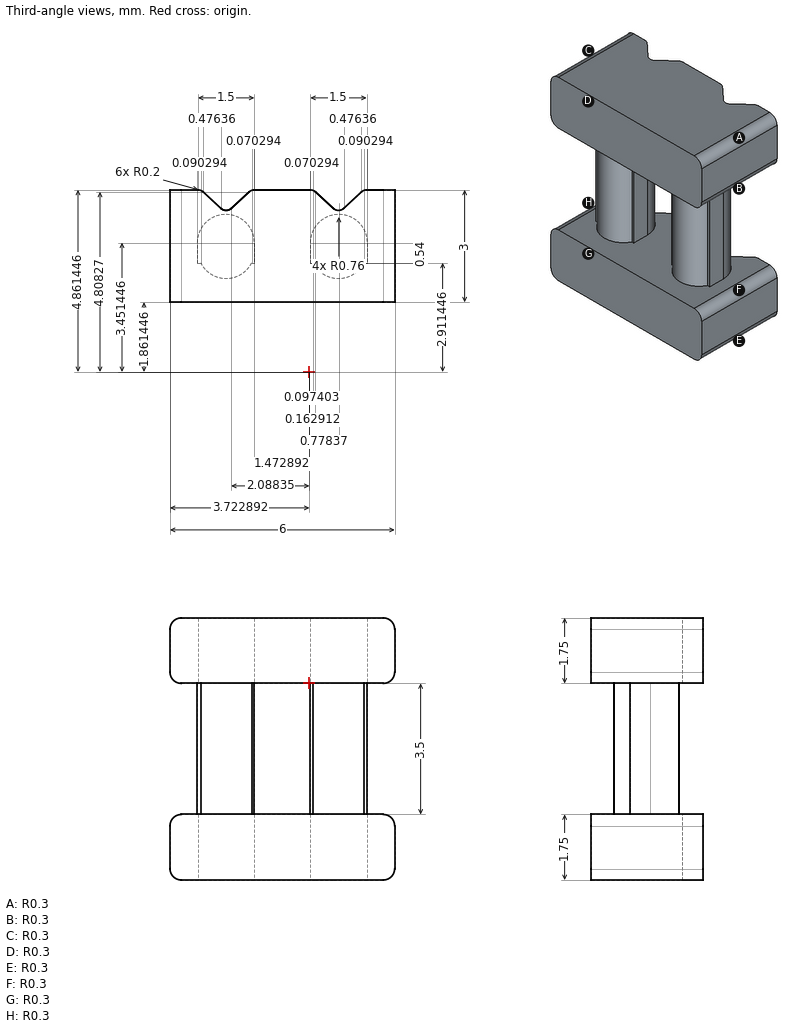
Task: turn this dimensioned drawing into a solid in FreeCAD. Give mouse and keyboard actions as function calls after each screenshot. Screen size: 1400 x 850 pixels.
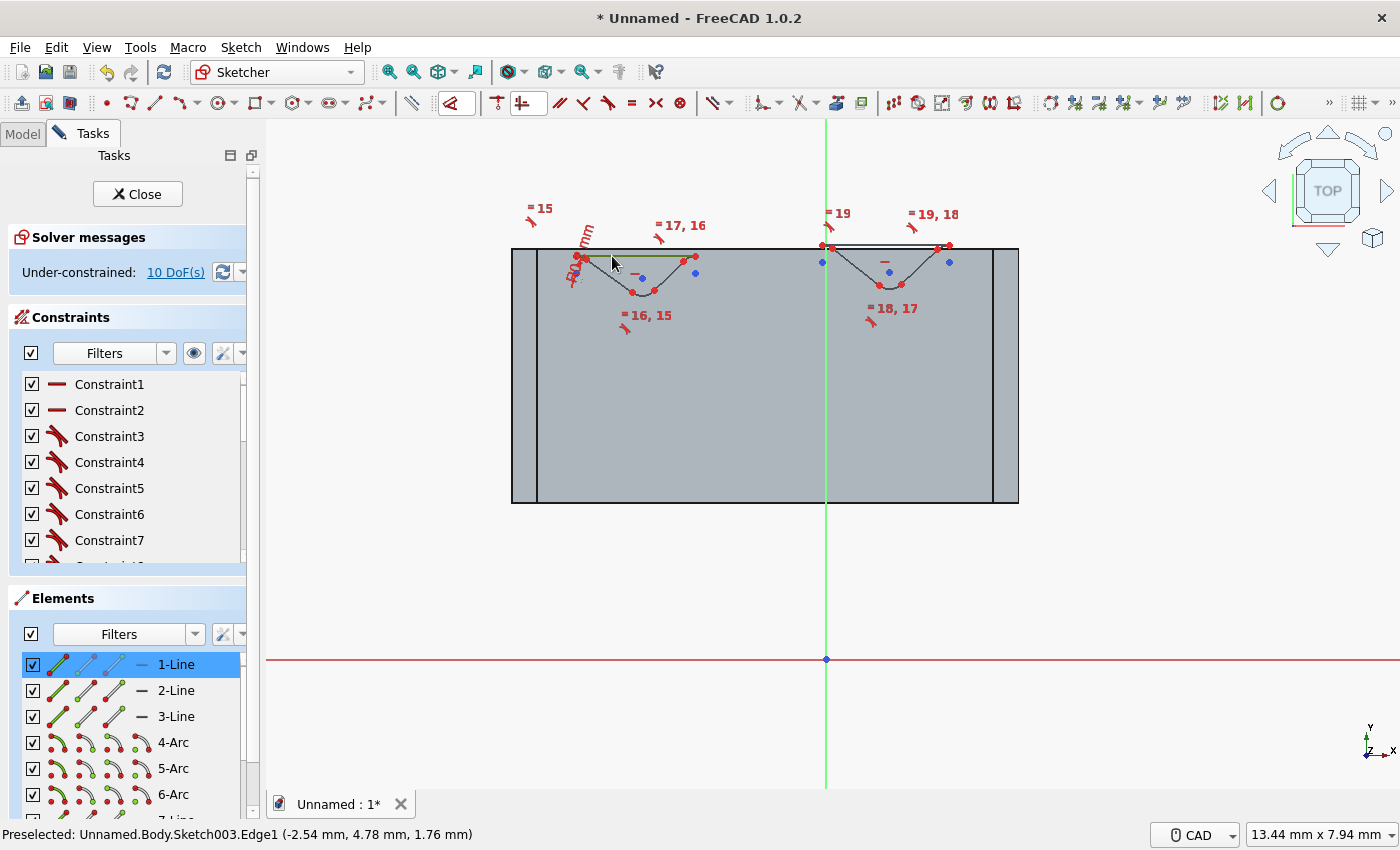
click(470, 104)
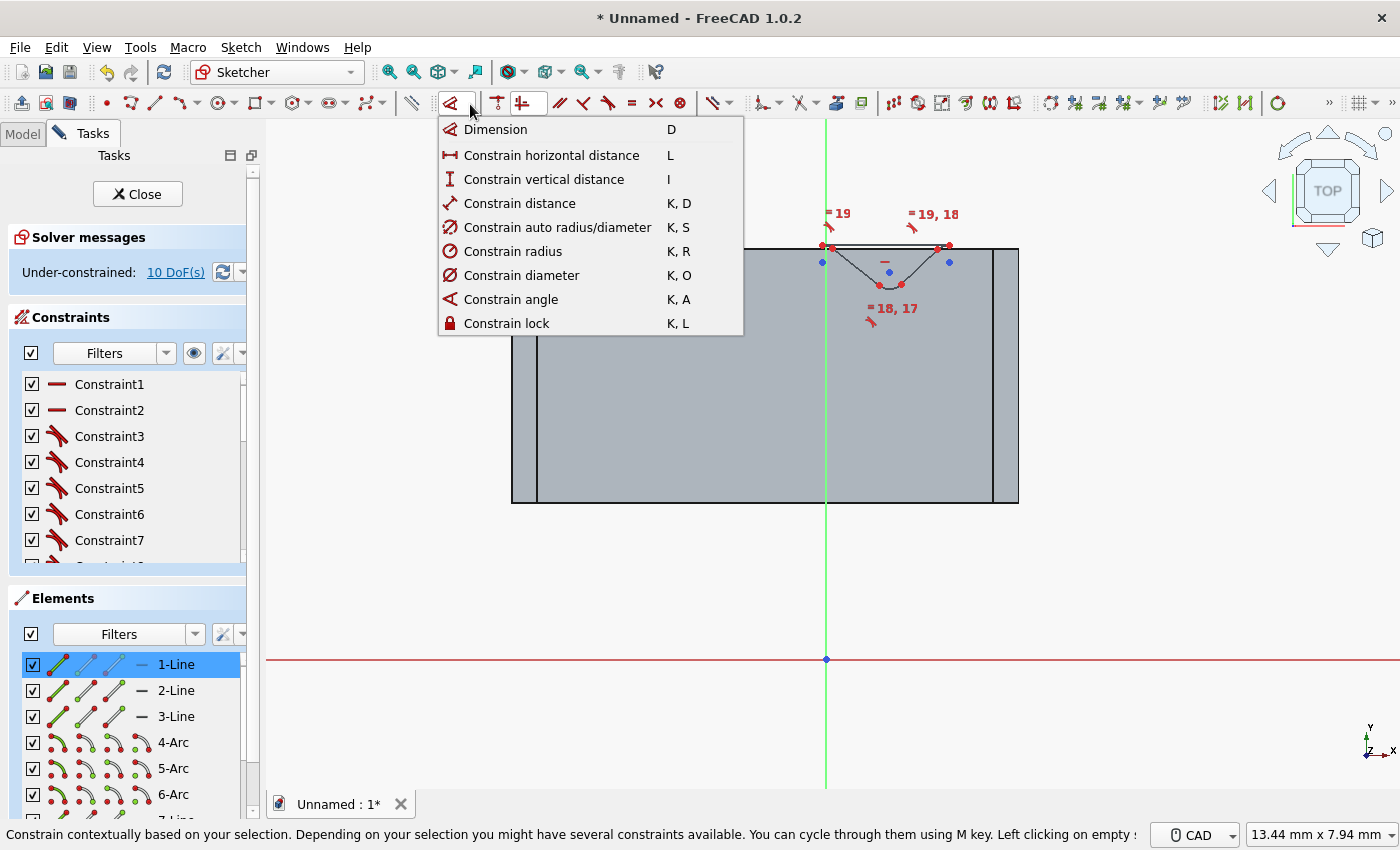
click(591, 155)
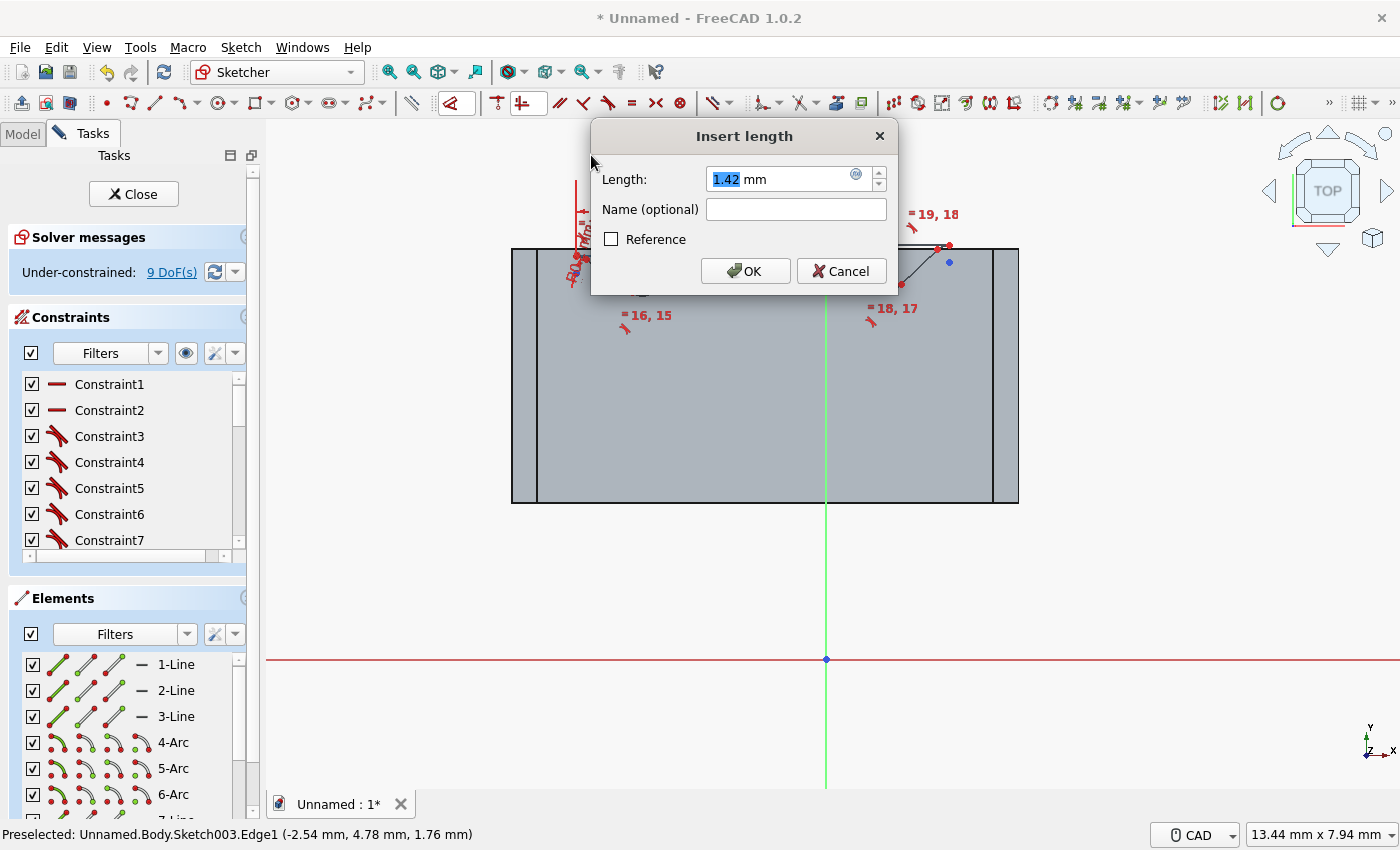
text(1.5)
key(Return)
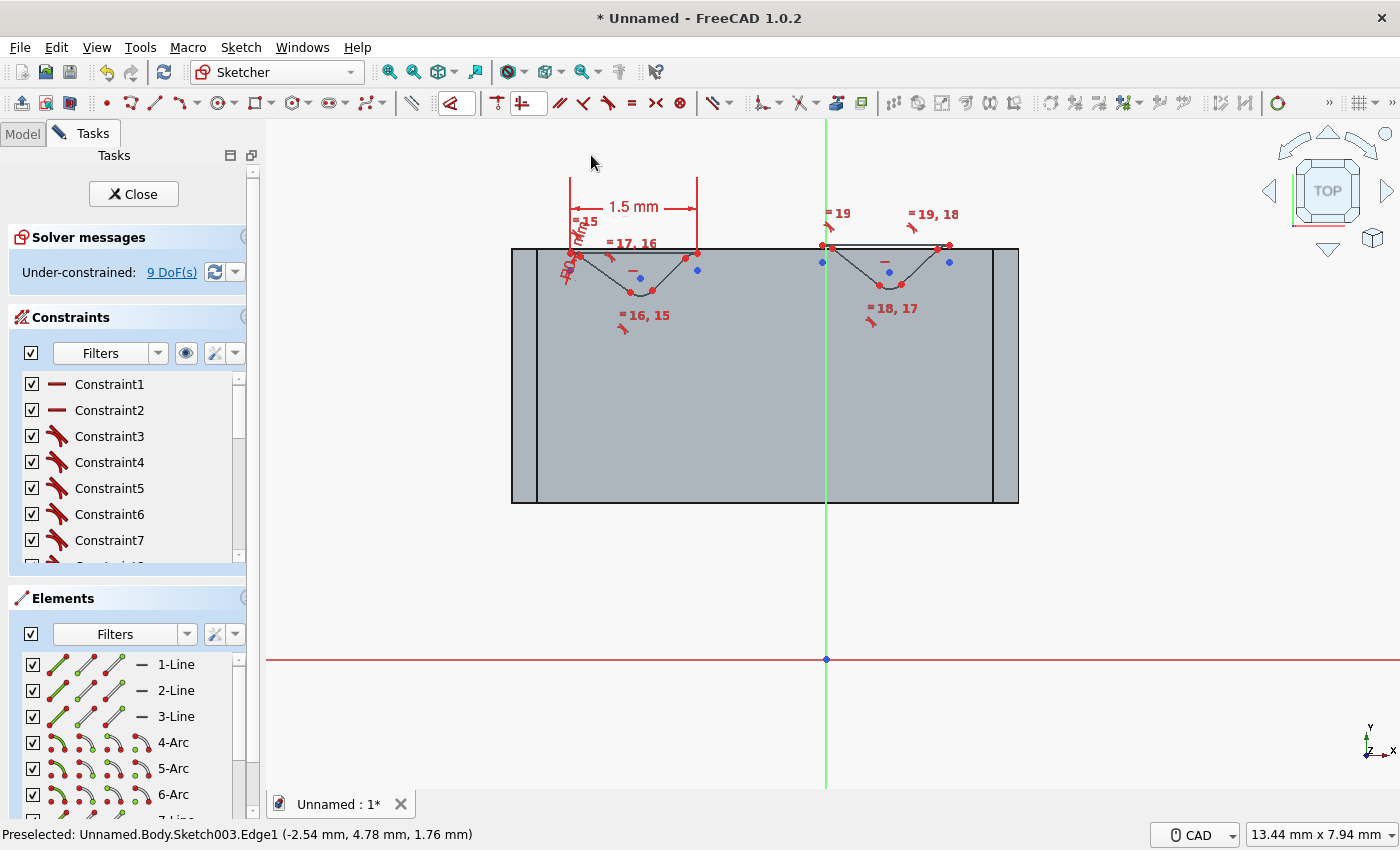
click(911, 245)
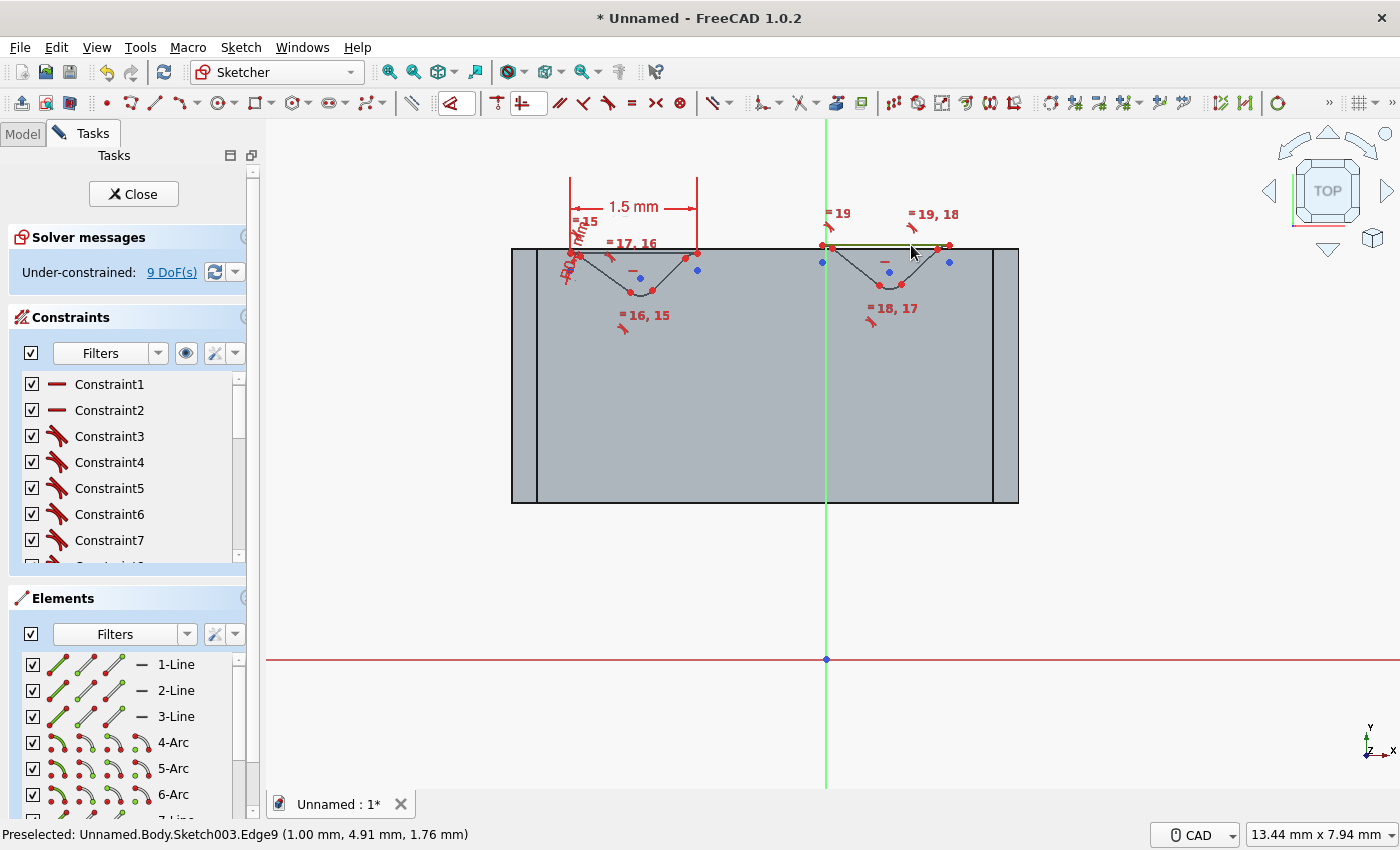
key(l)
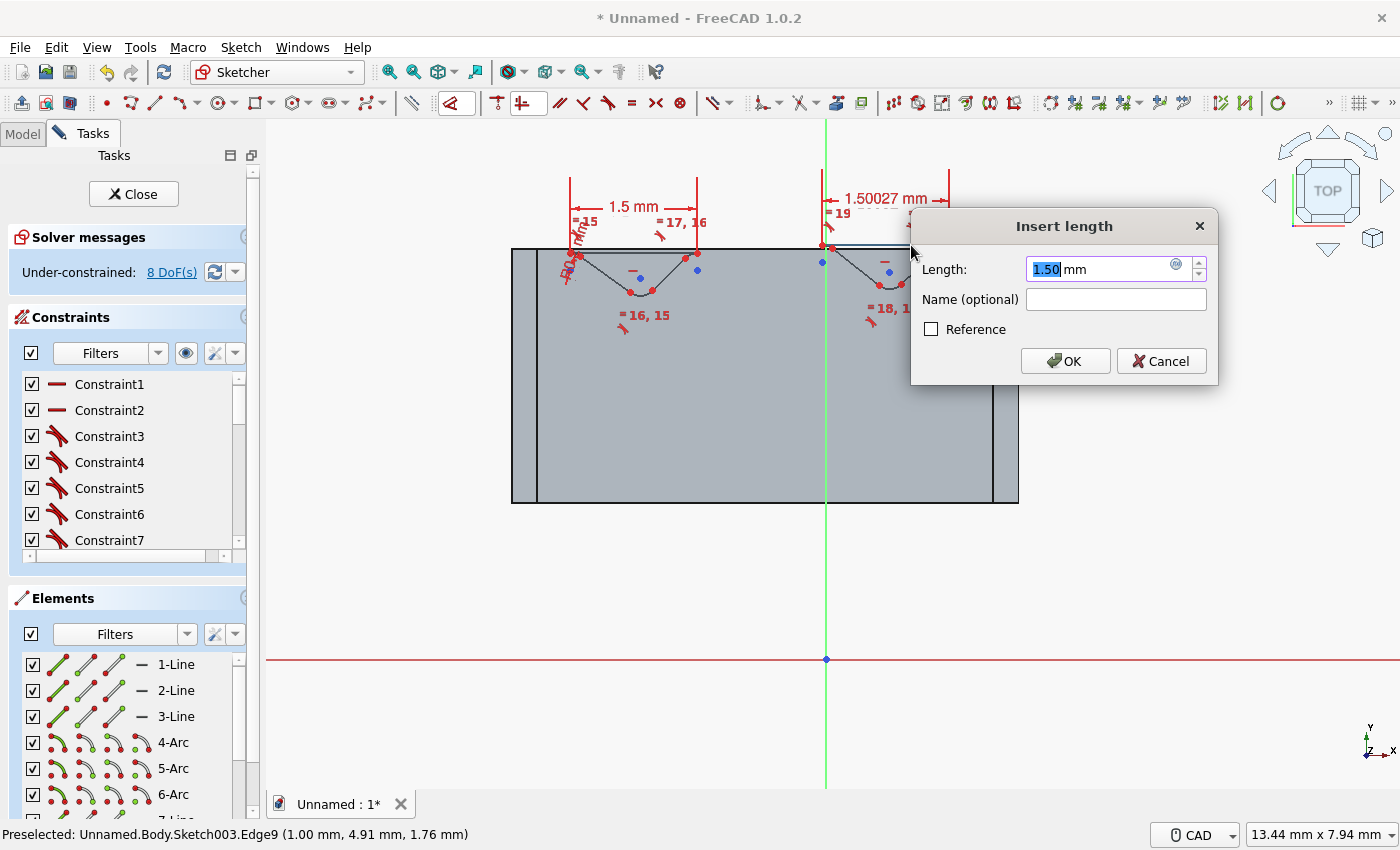
text(1.5)
key(Return)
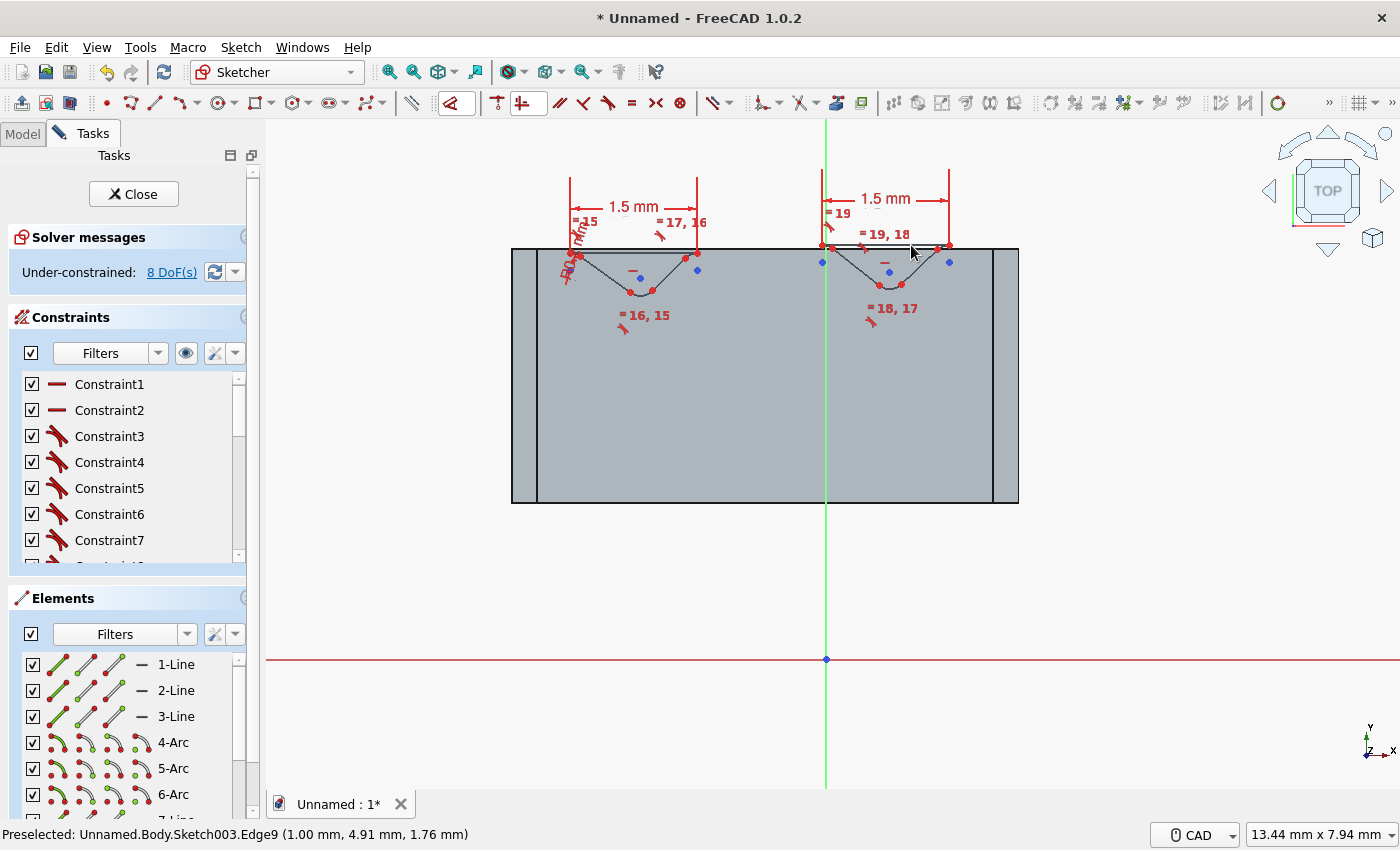
click(652, 291)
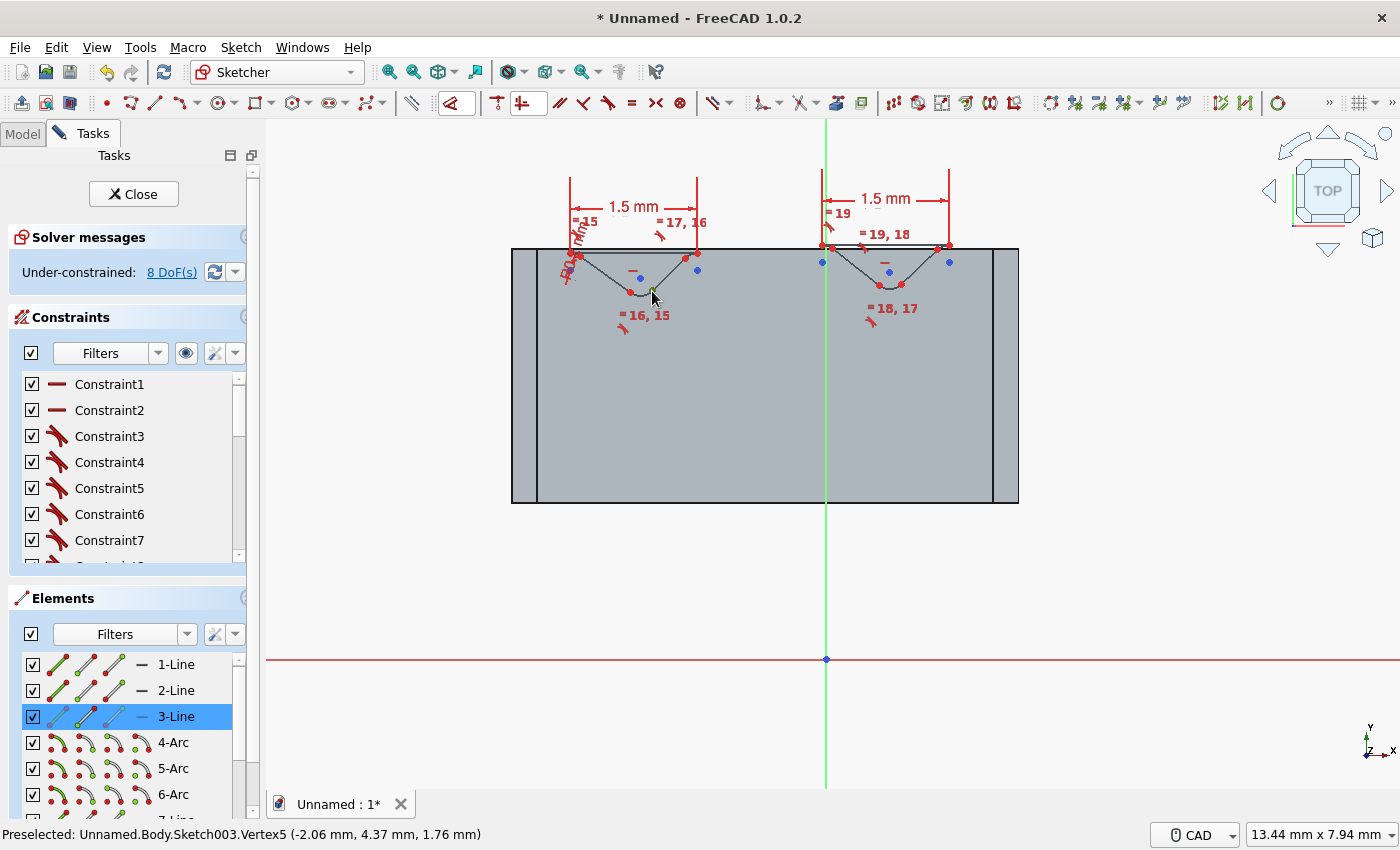
click(470, 104)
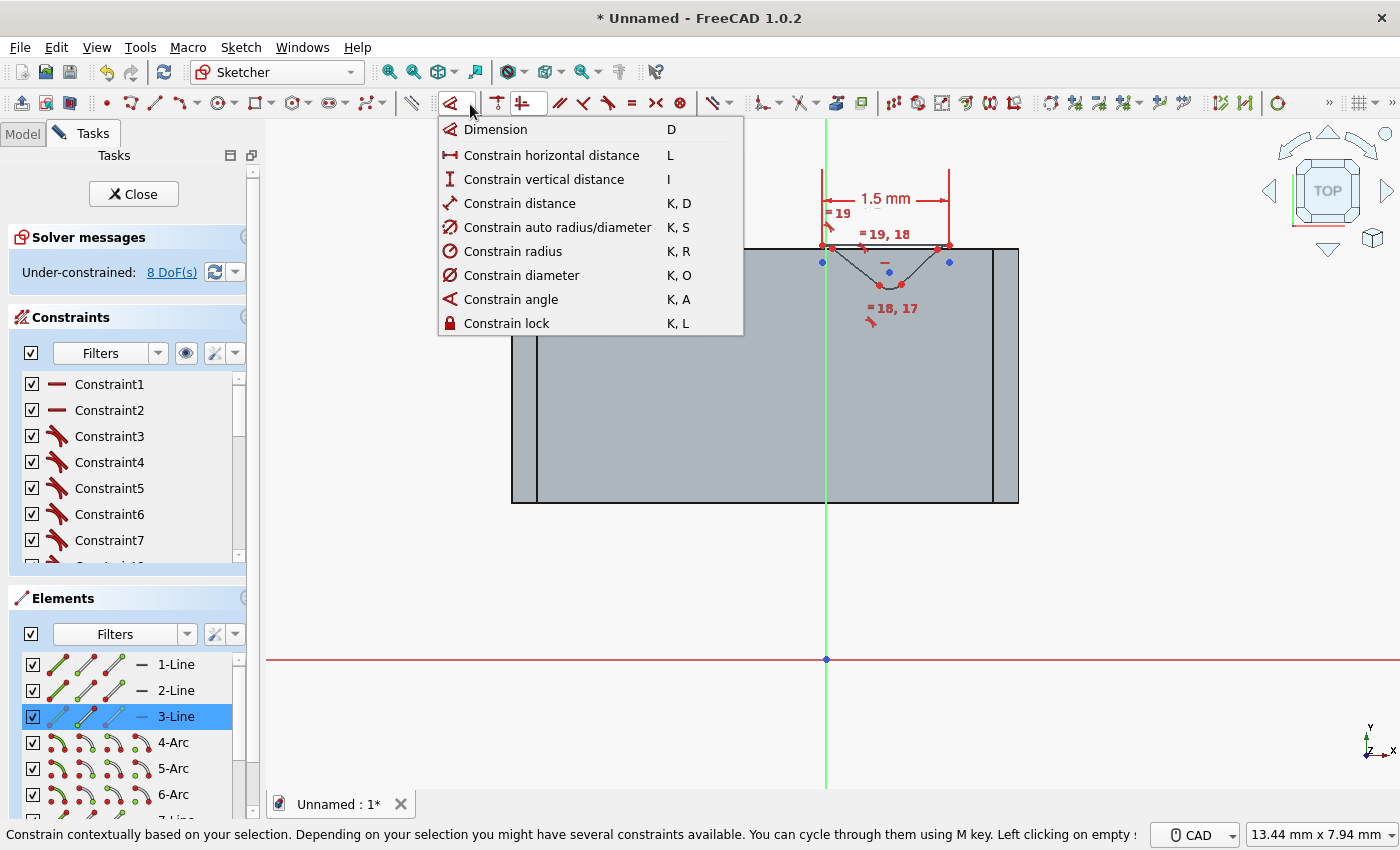
click(591, 155)